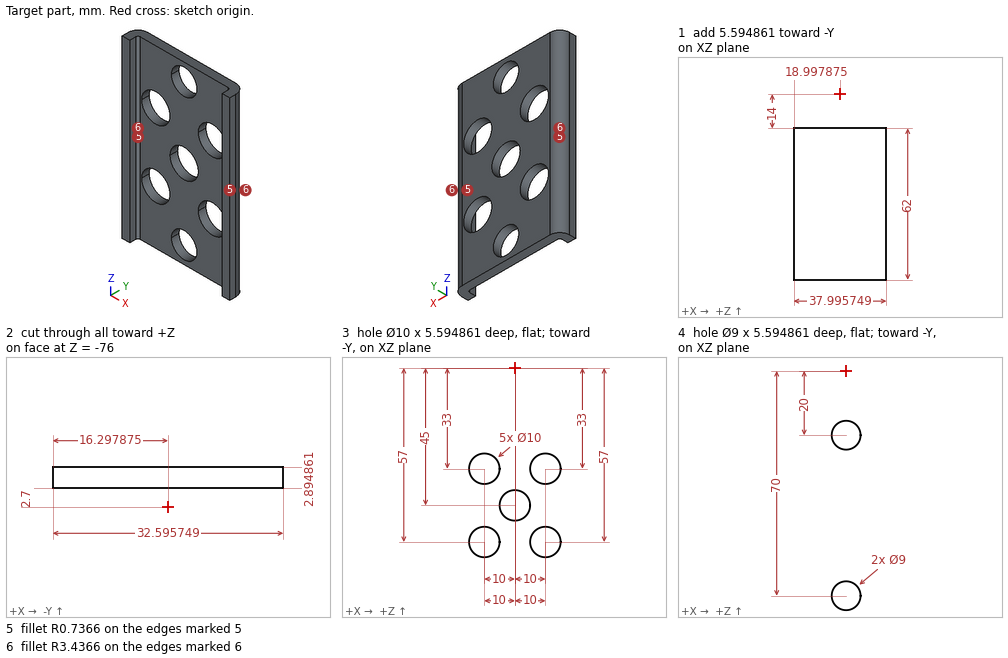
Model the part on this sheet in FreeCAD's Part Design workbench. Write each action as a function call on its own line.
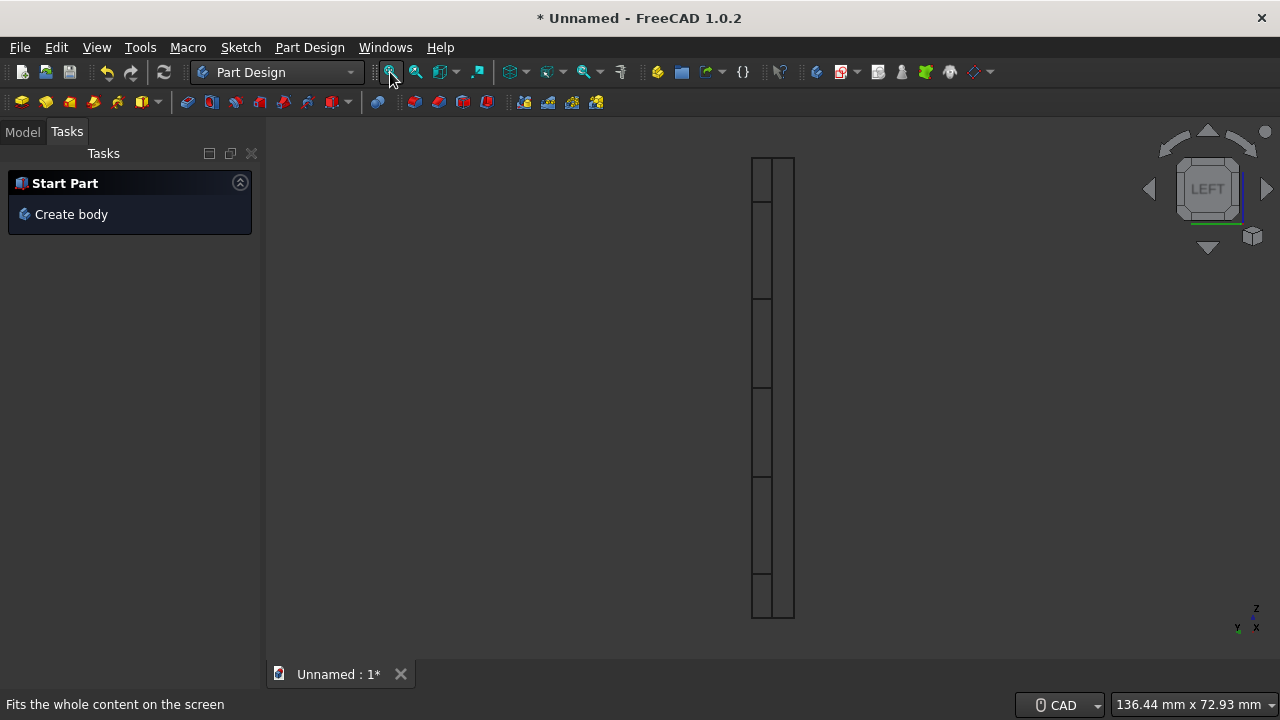
key(0)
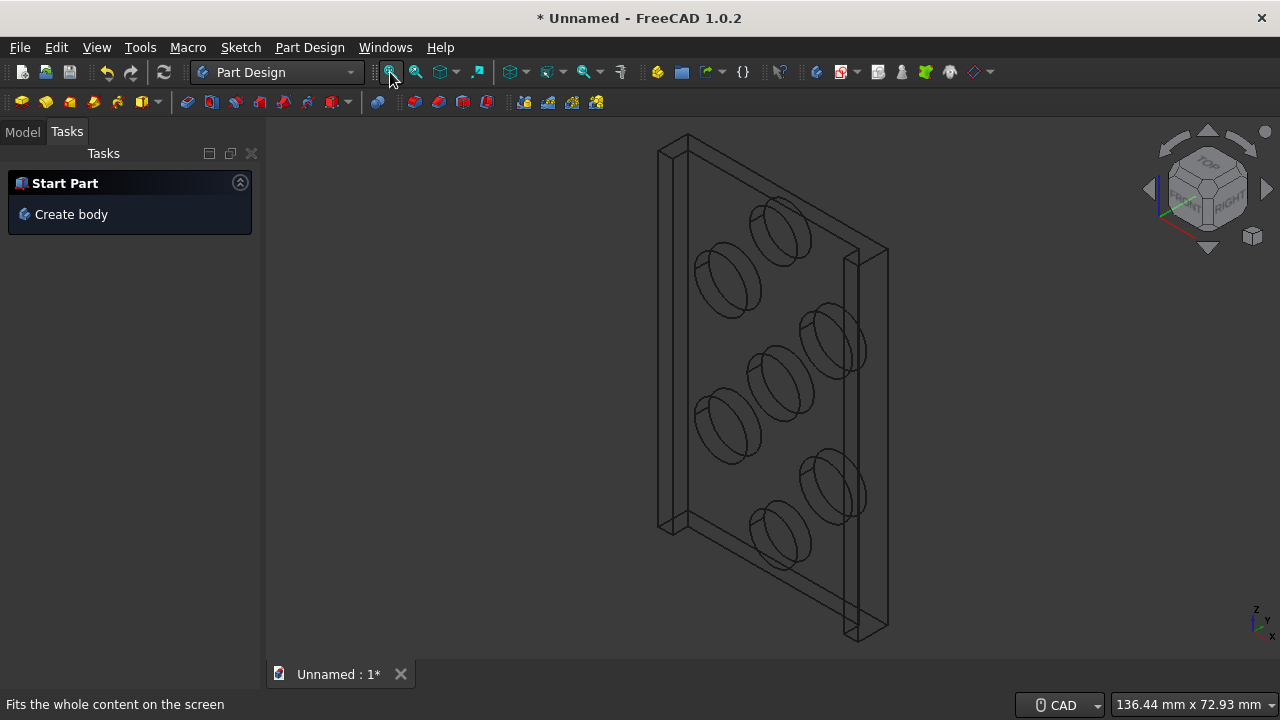
click(688, 337)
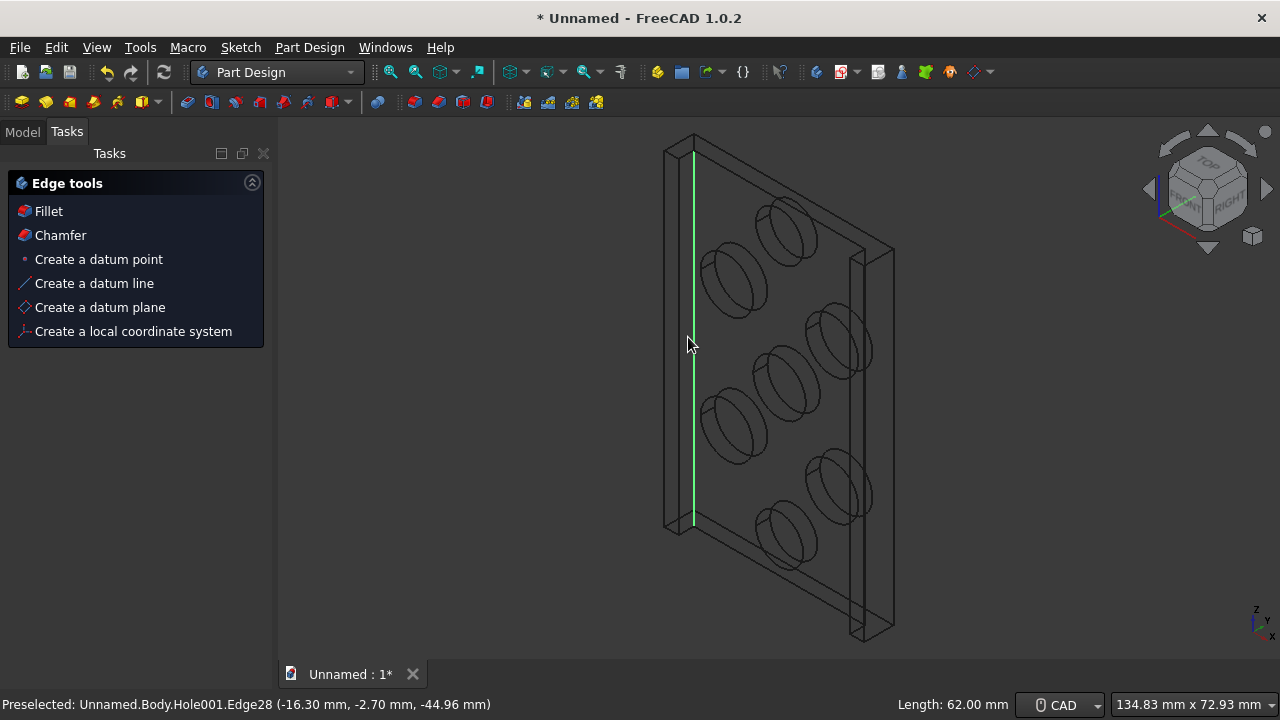
scroll(865, 436, up, 6)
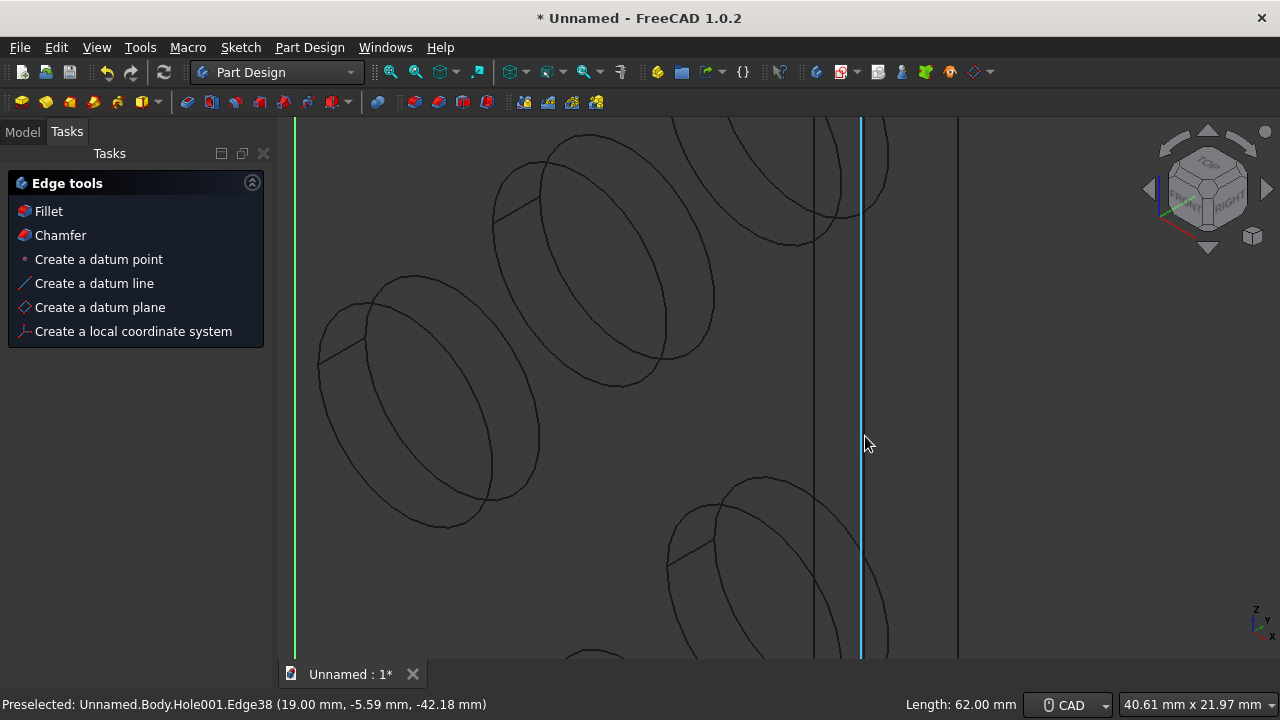
click(392, 72)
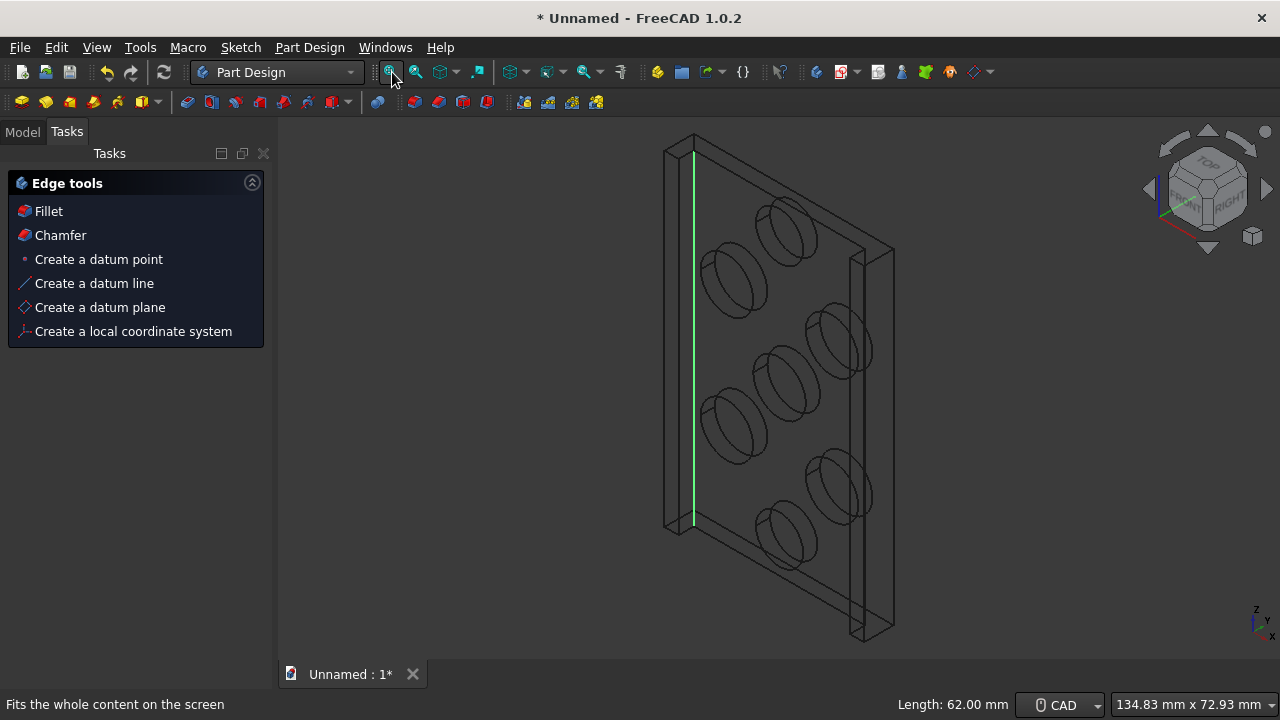
key(2)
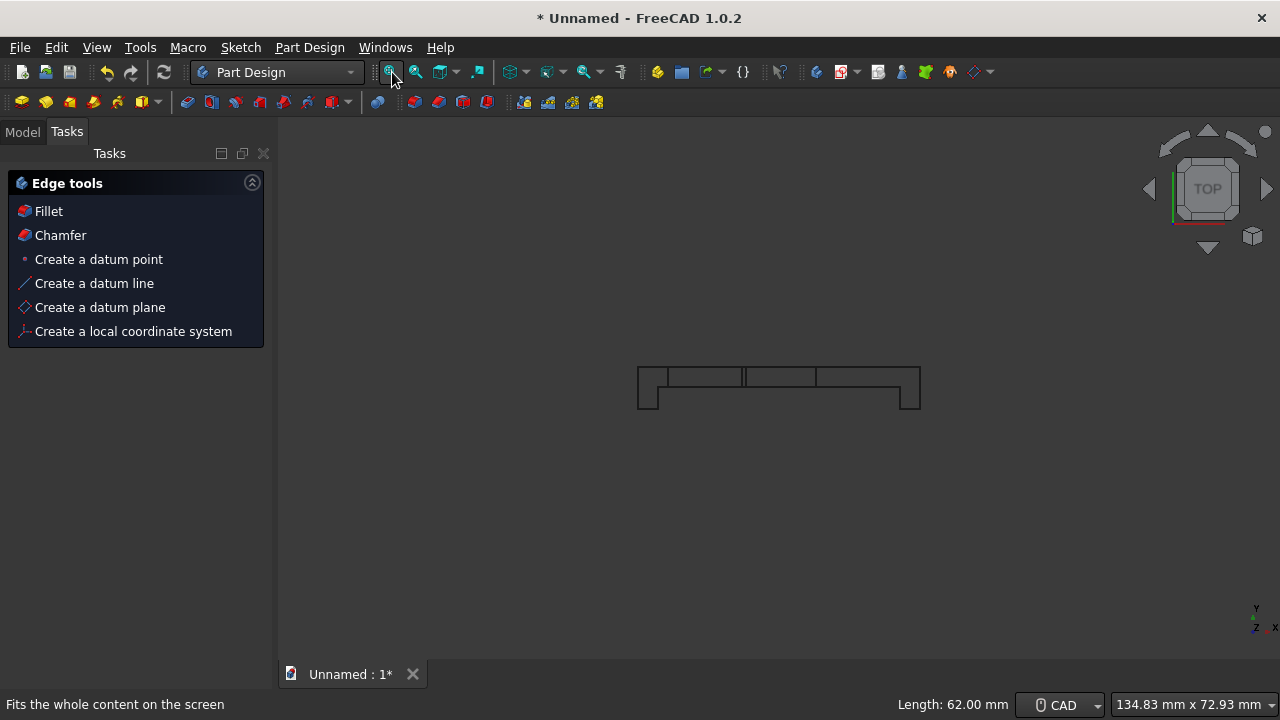
key(v)
key(f)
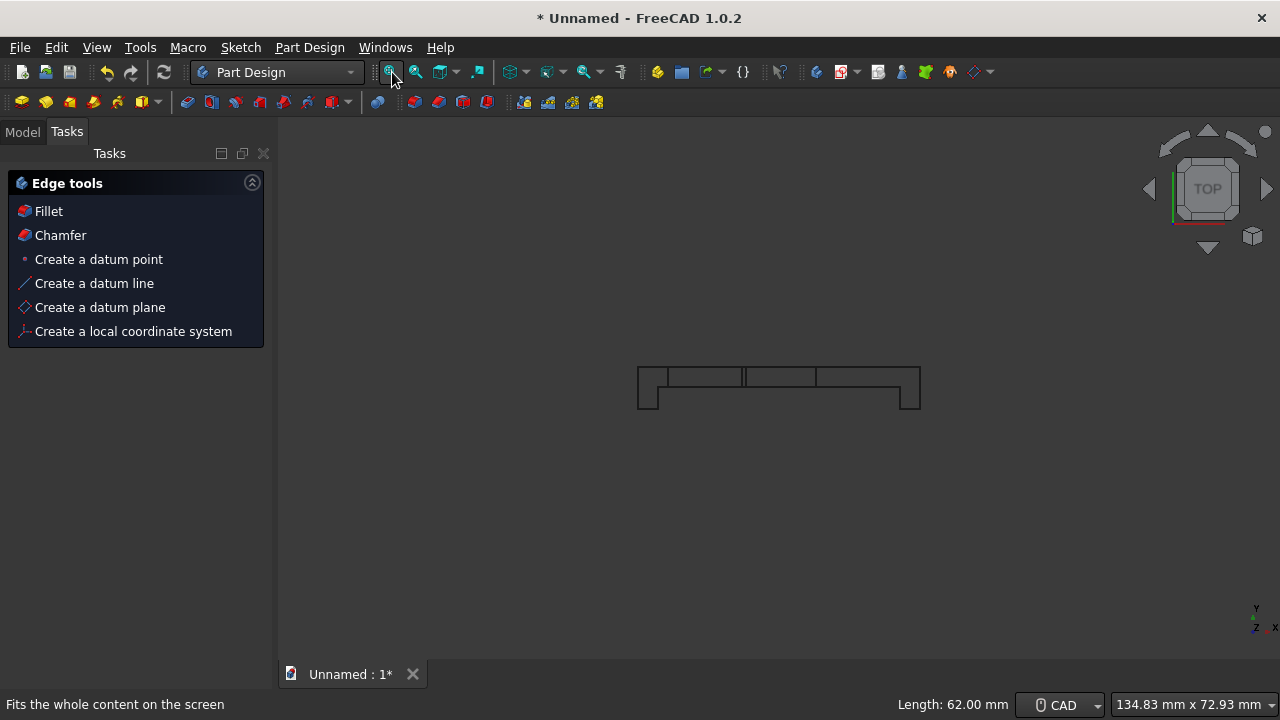
scroll(900, 386, up, 6)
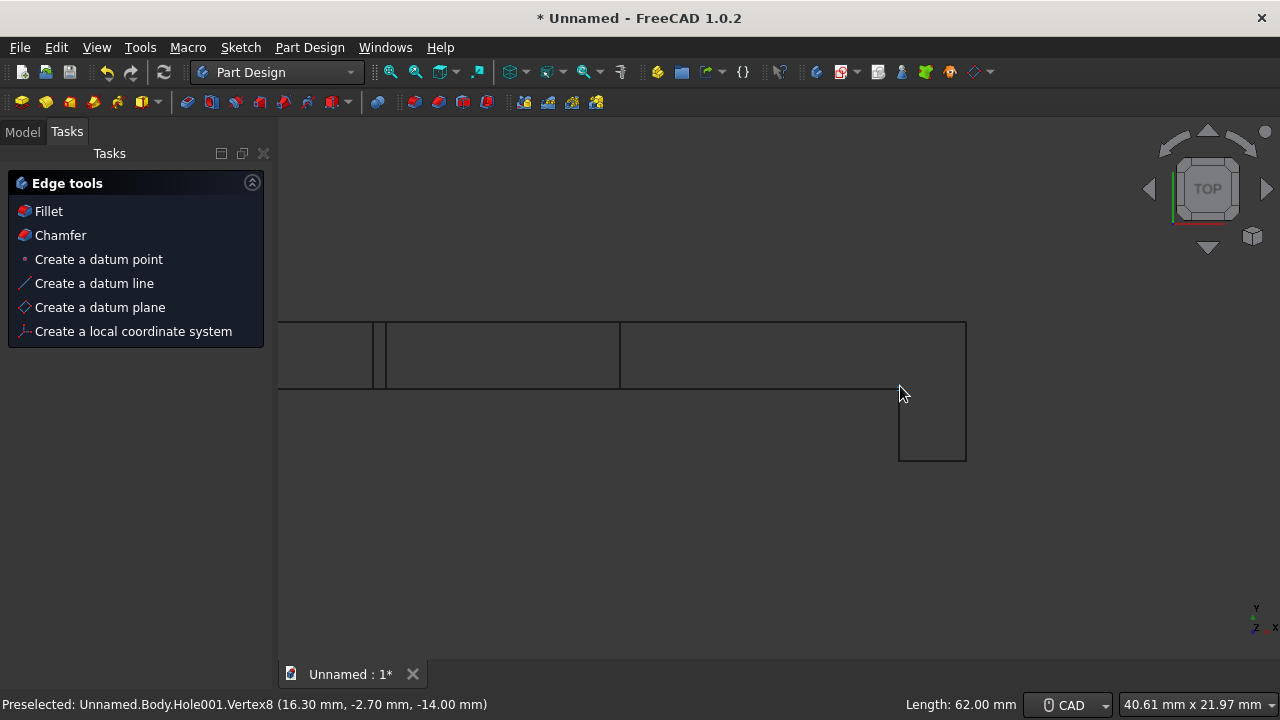
click(392, 72)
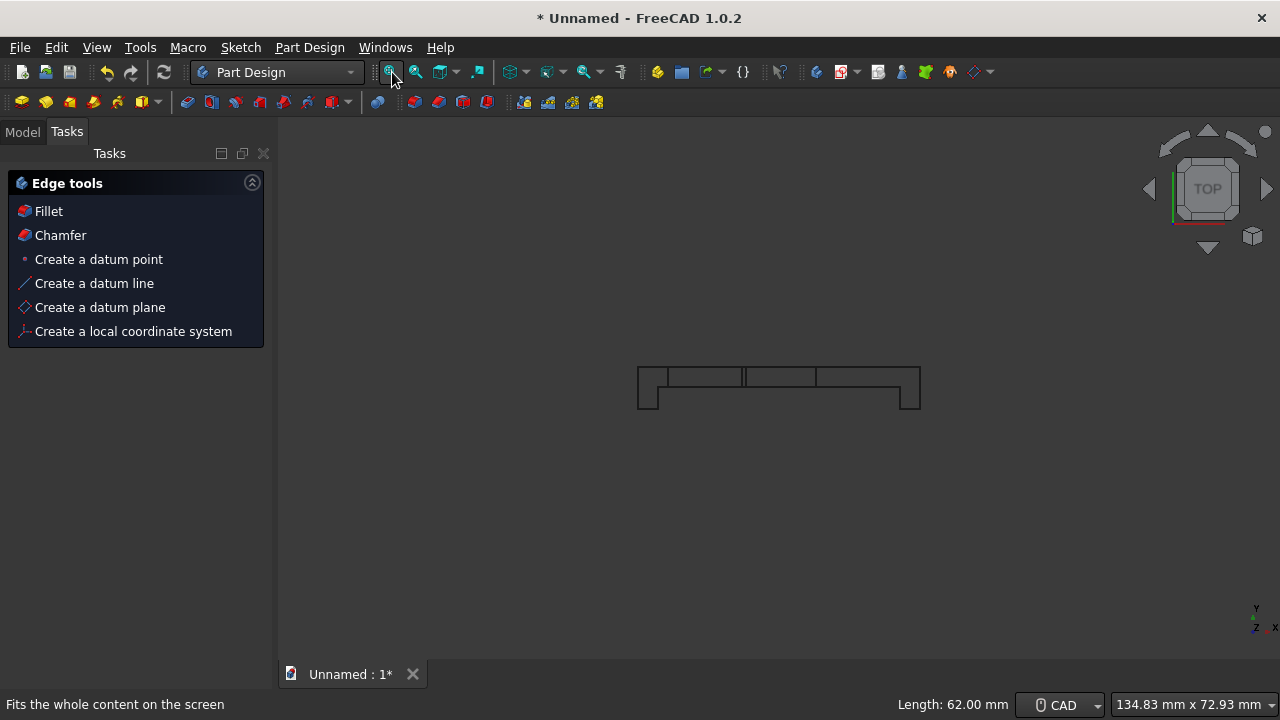
key(1)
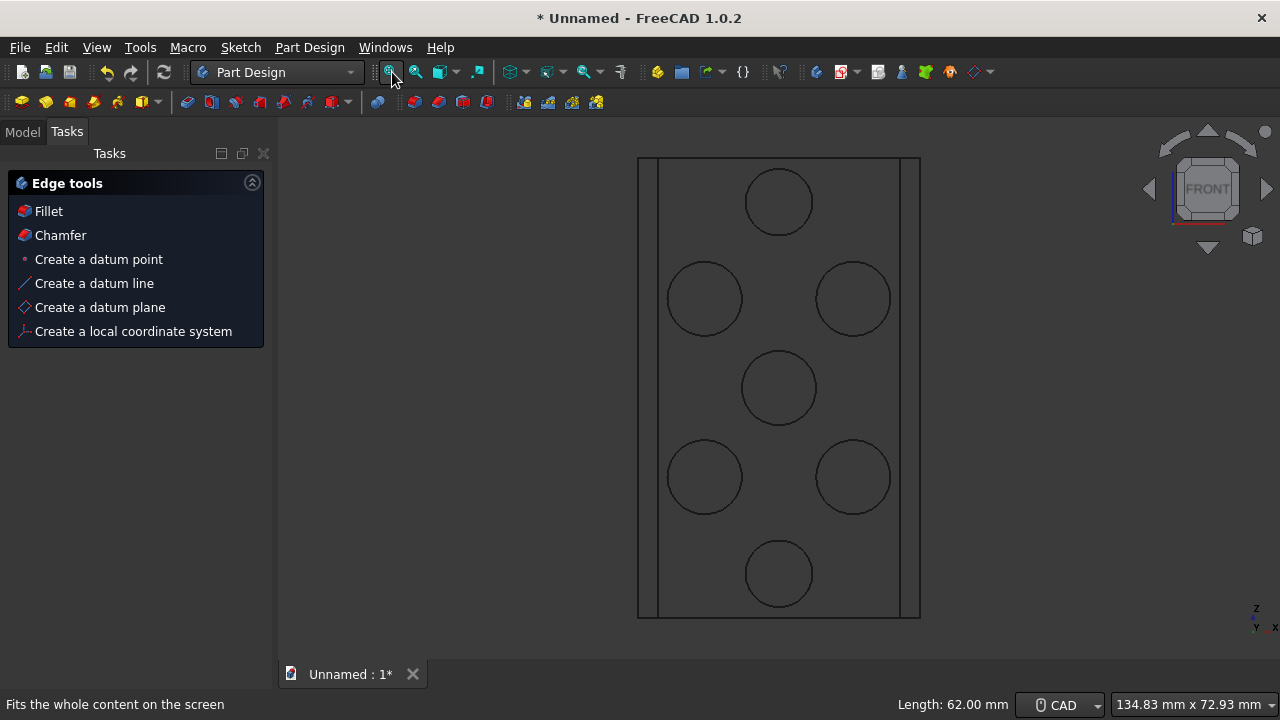
scroll(900, 387, up, 6)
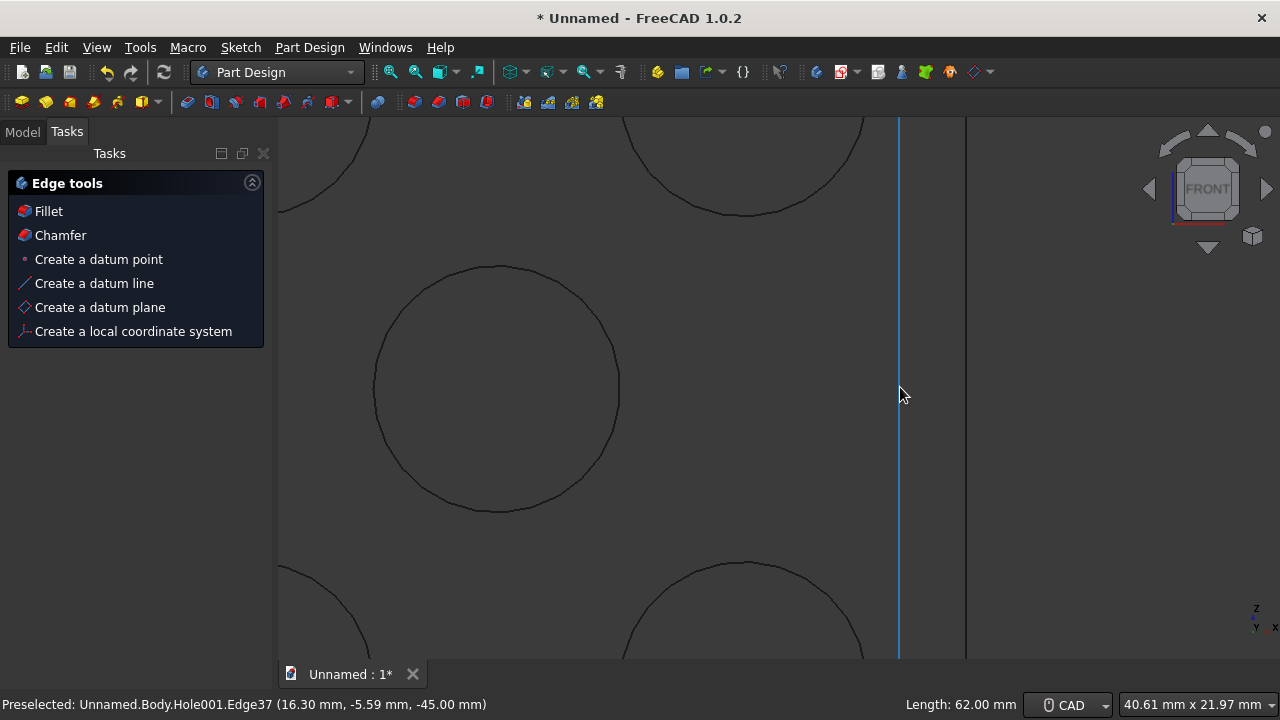
key(v)
key(f)